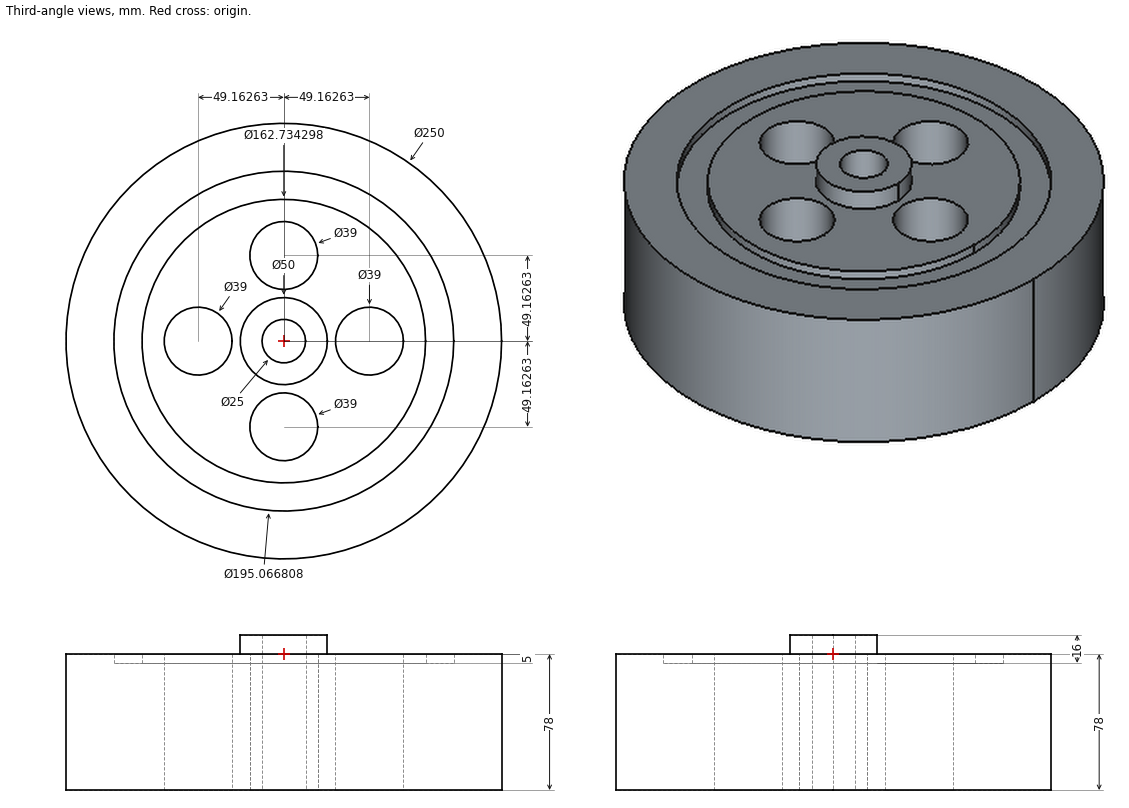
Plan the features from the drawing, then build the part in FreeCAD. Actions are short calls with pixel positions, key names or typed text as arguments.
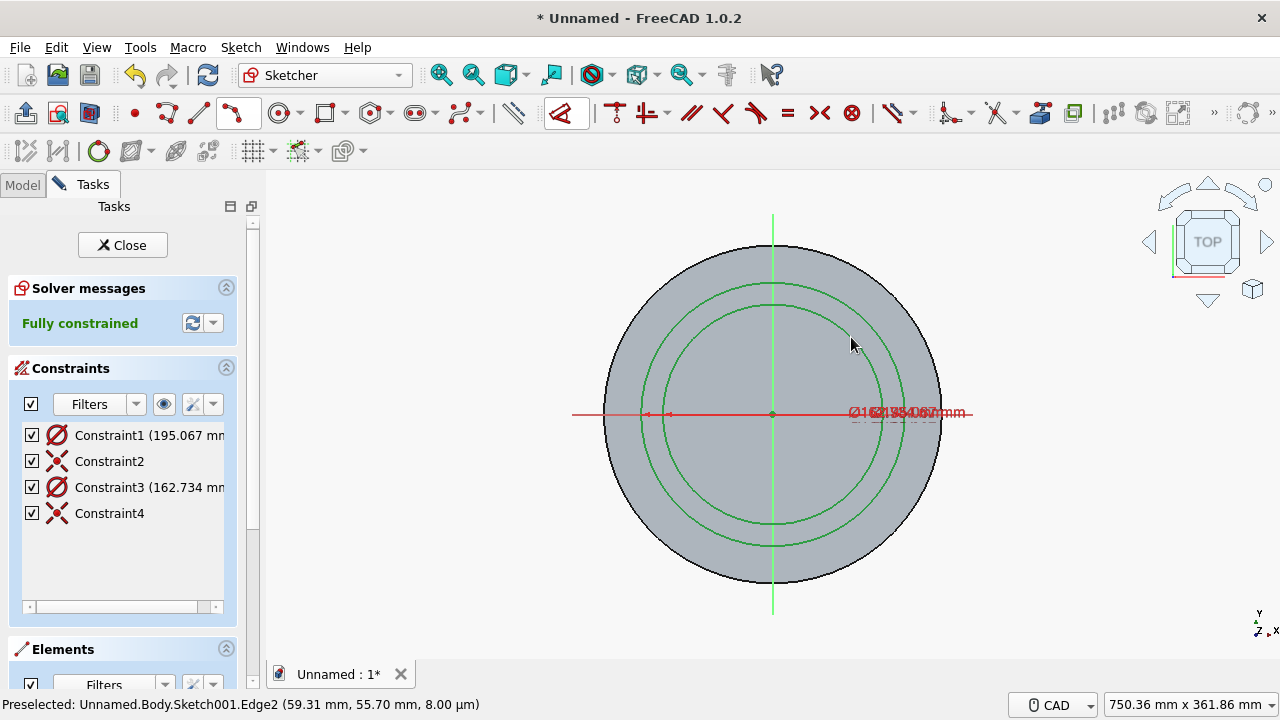
click(123, 245)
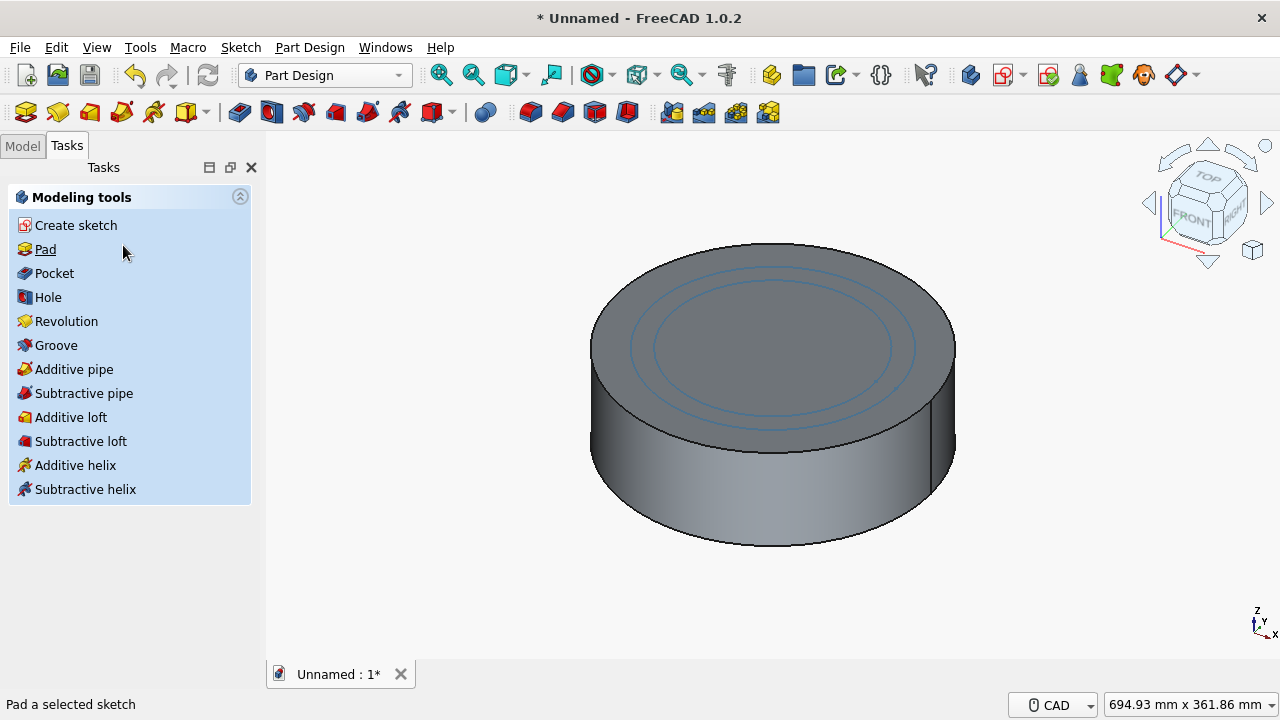
click(240, 112)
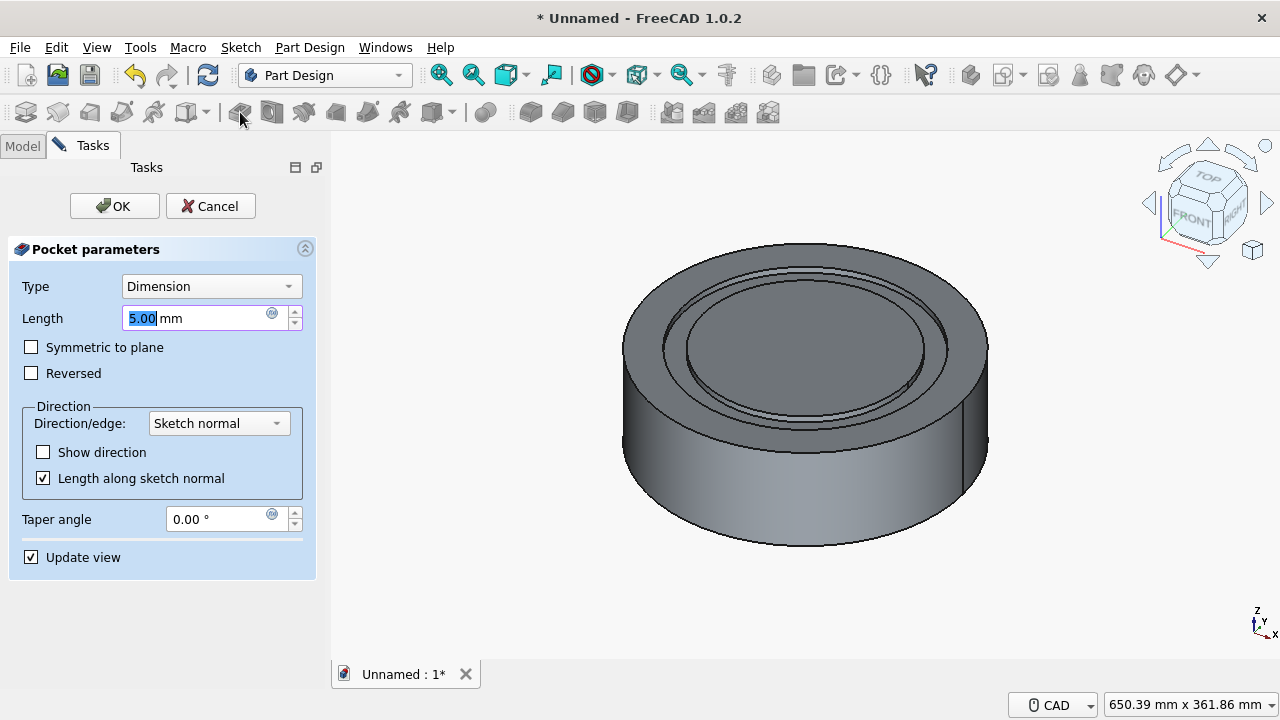
text(5)
key(Tab)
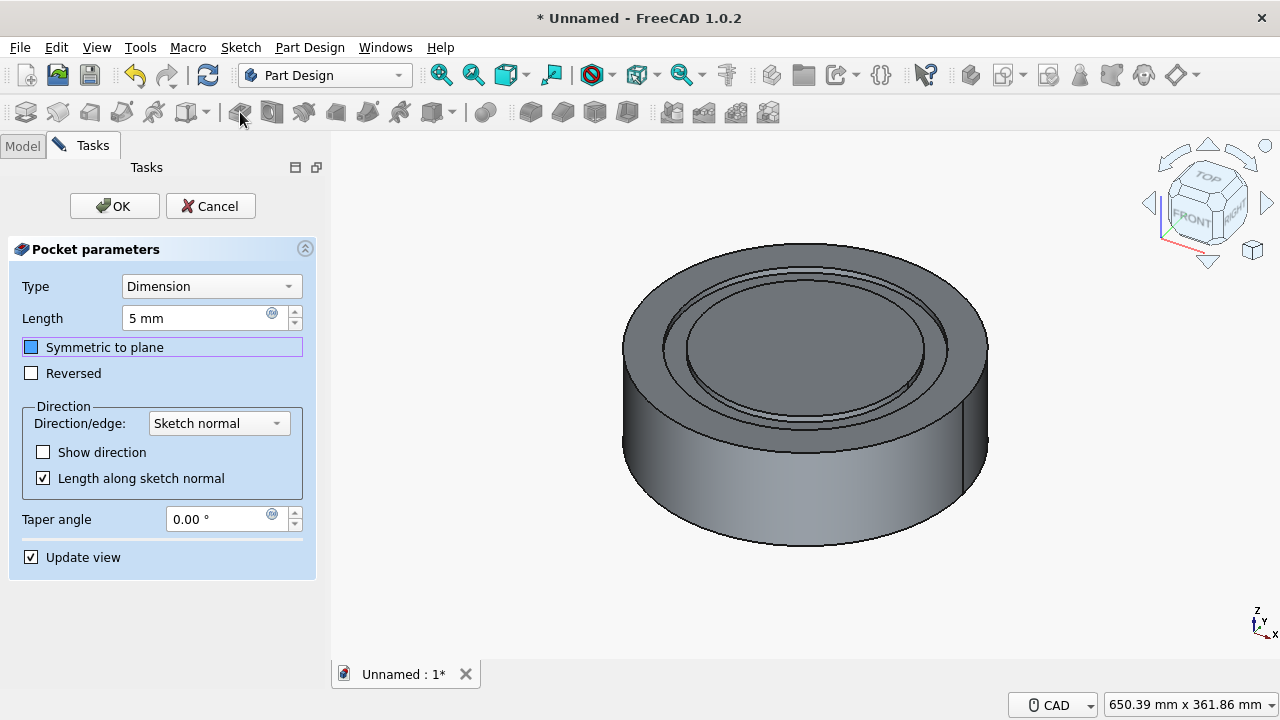
click(115, 206)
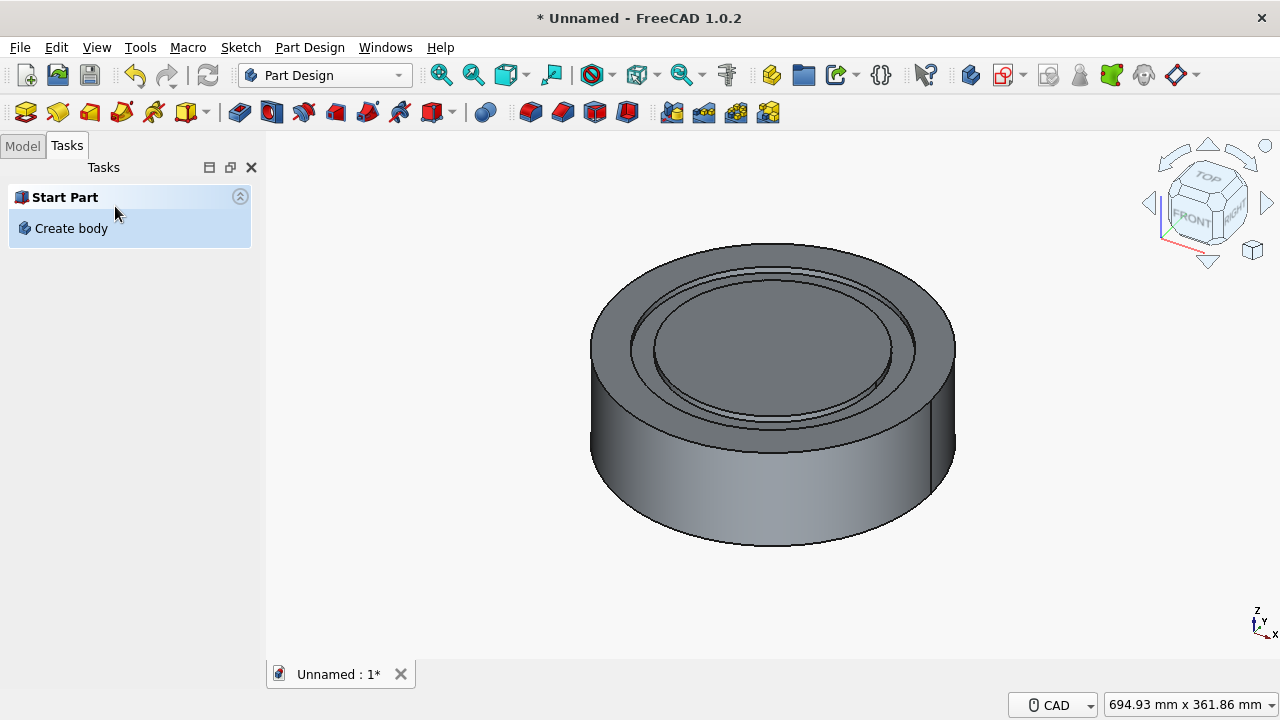
click(1004, 76)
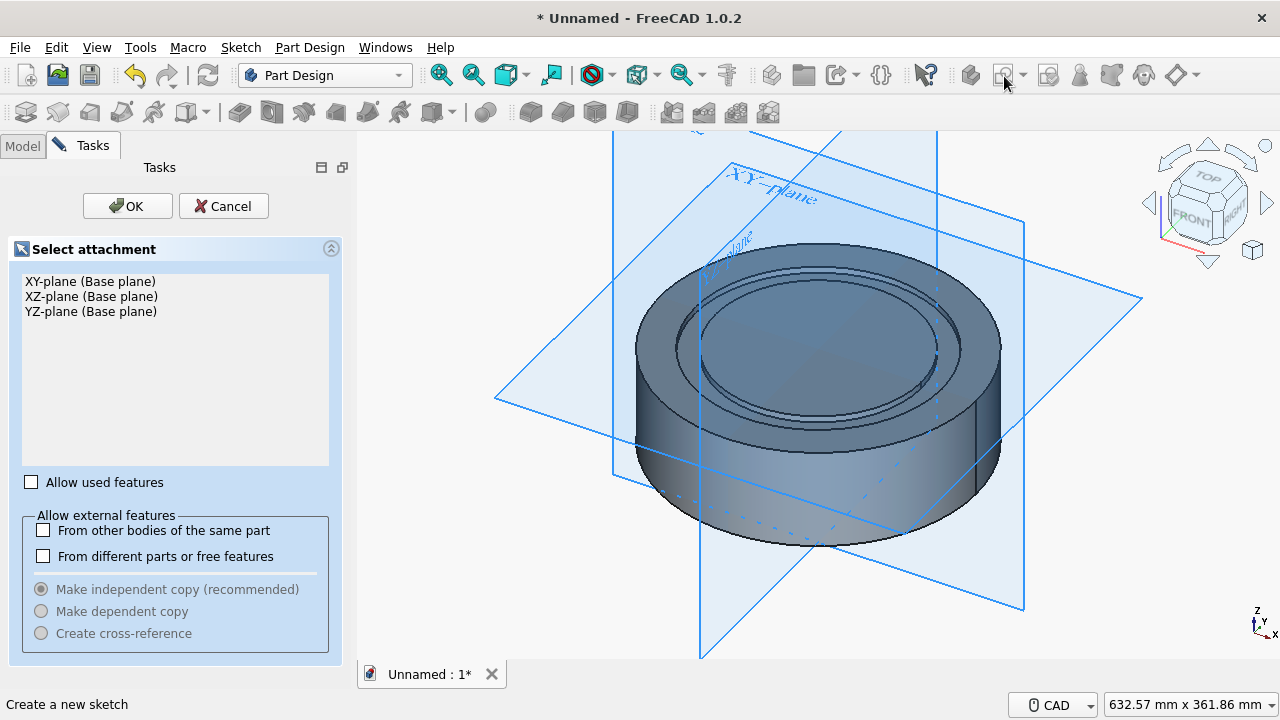
click(82, 282)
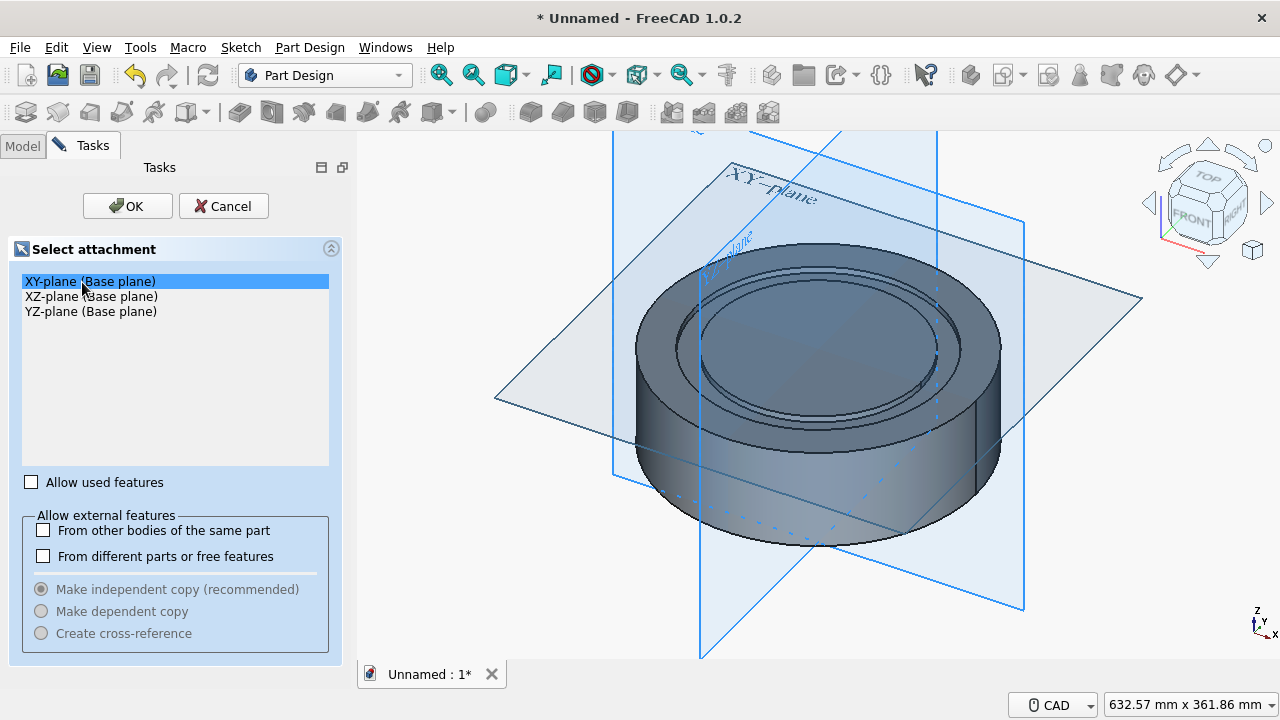
click(128, 206)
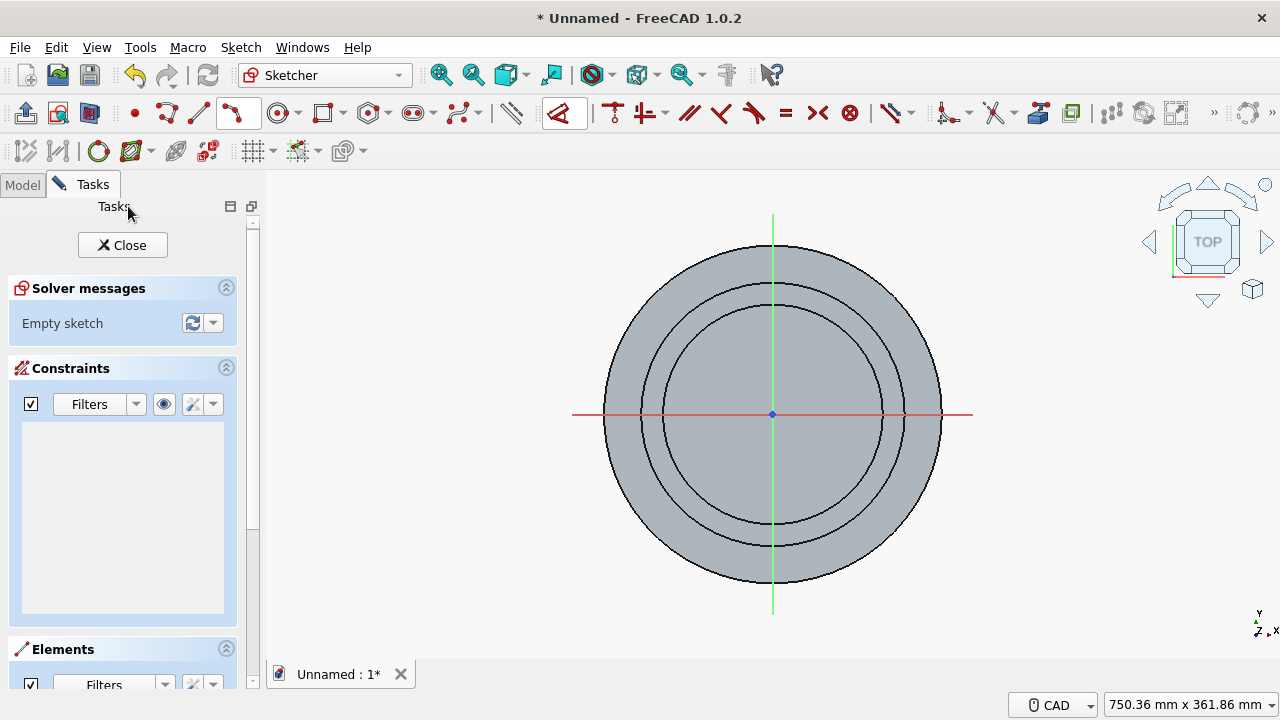
scroll(802, 348, up, 6)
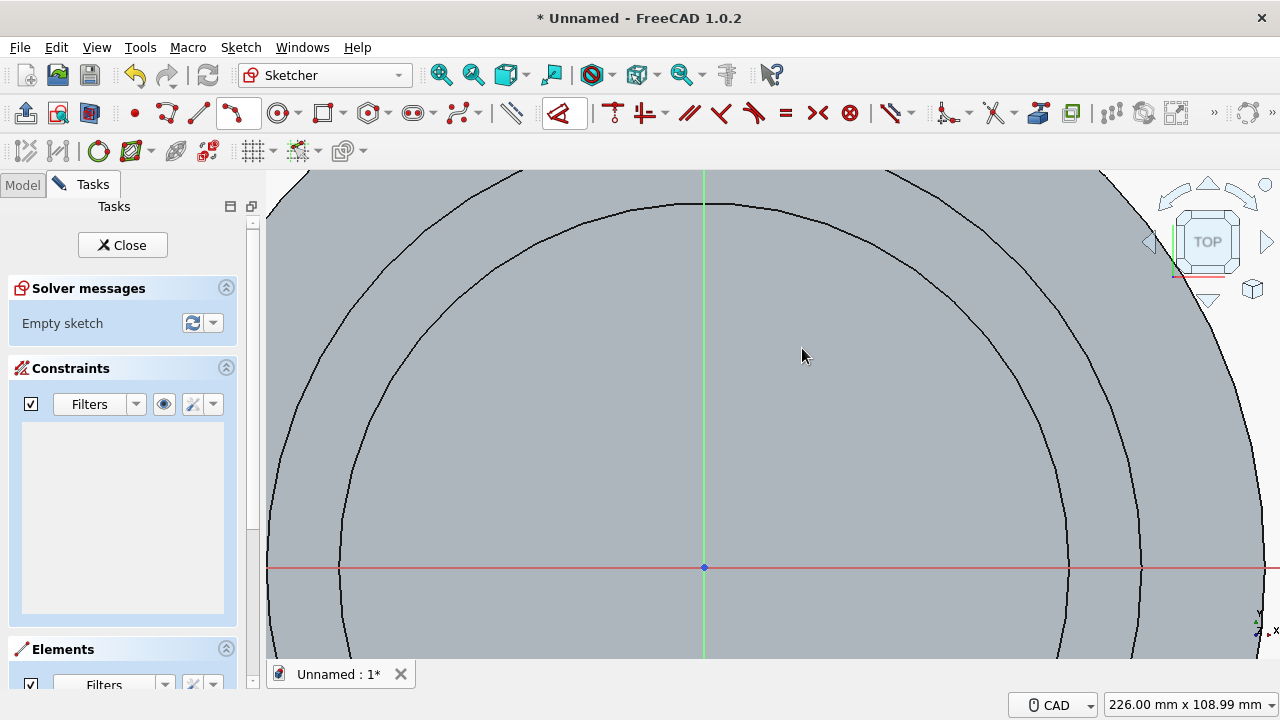
click(278, 114)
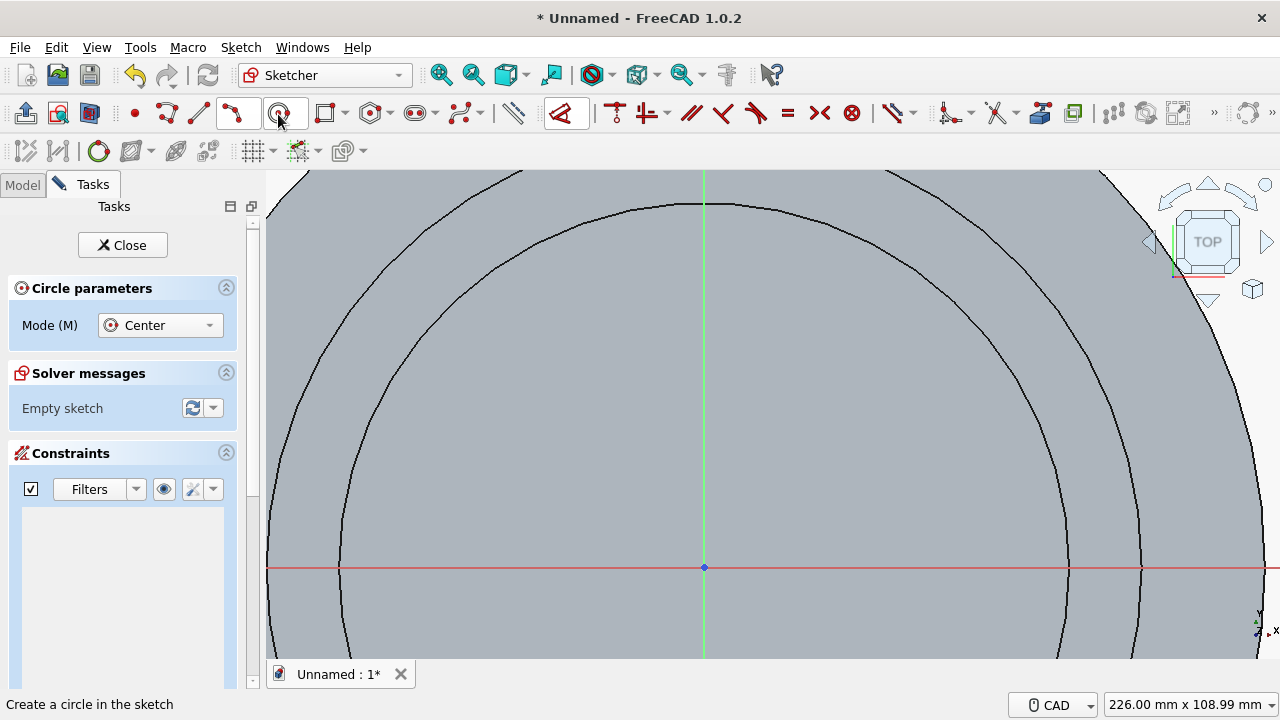
click(704, 347)
move(766, 286)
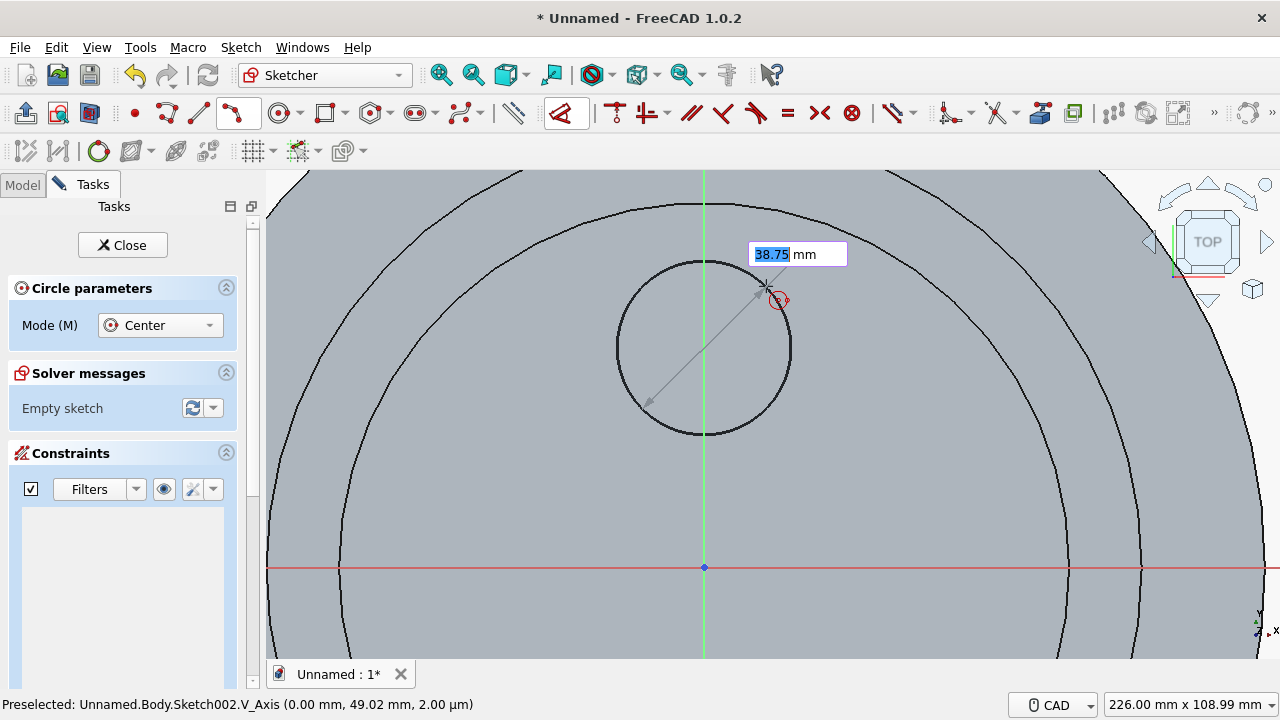
text(39)
key(Return)
key(Escape)